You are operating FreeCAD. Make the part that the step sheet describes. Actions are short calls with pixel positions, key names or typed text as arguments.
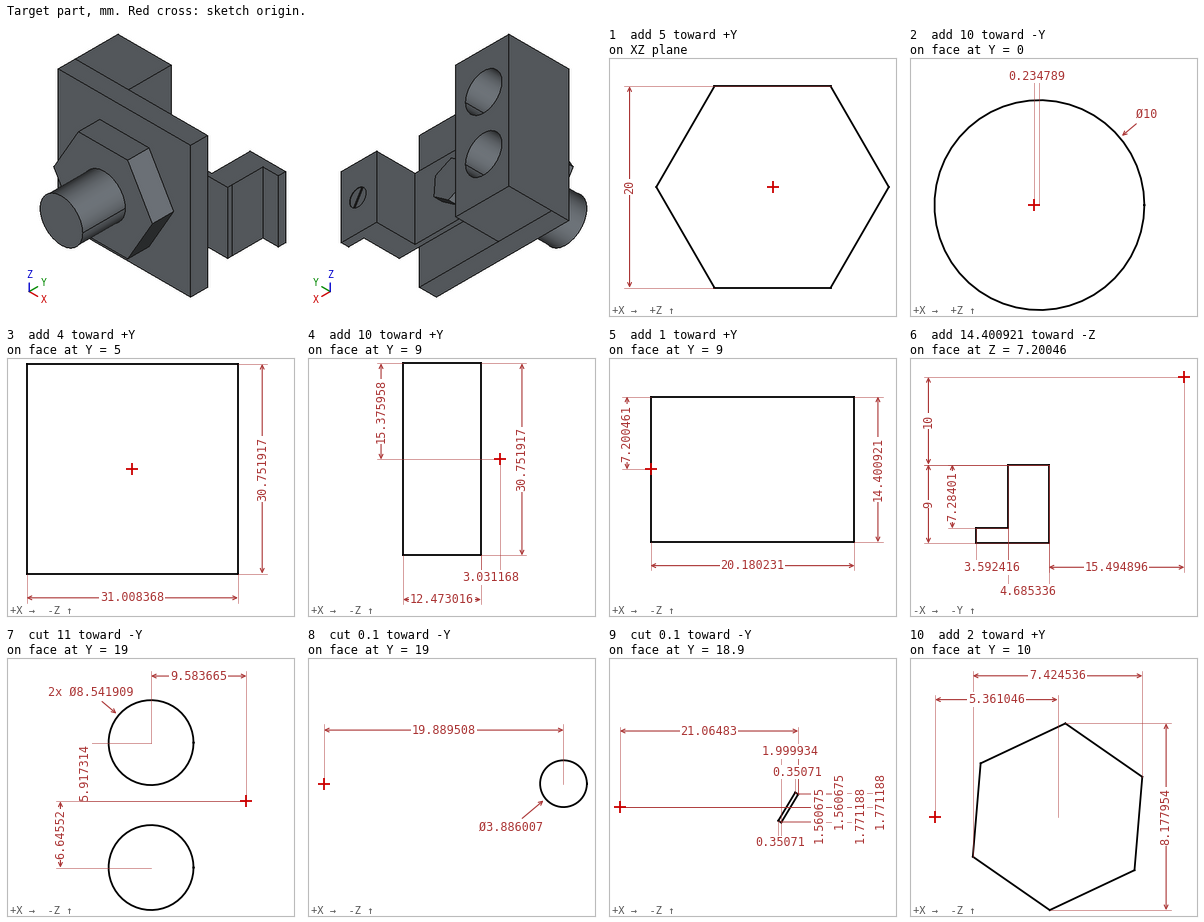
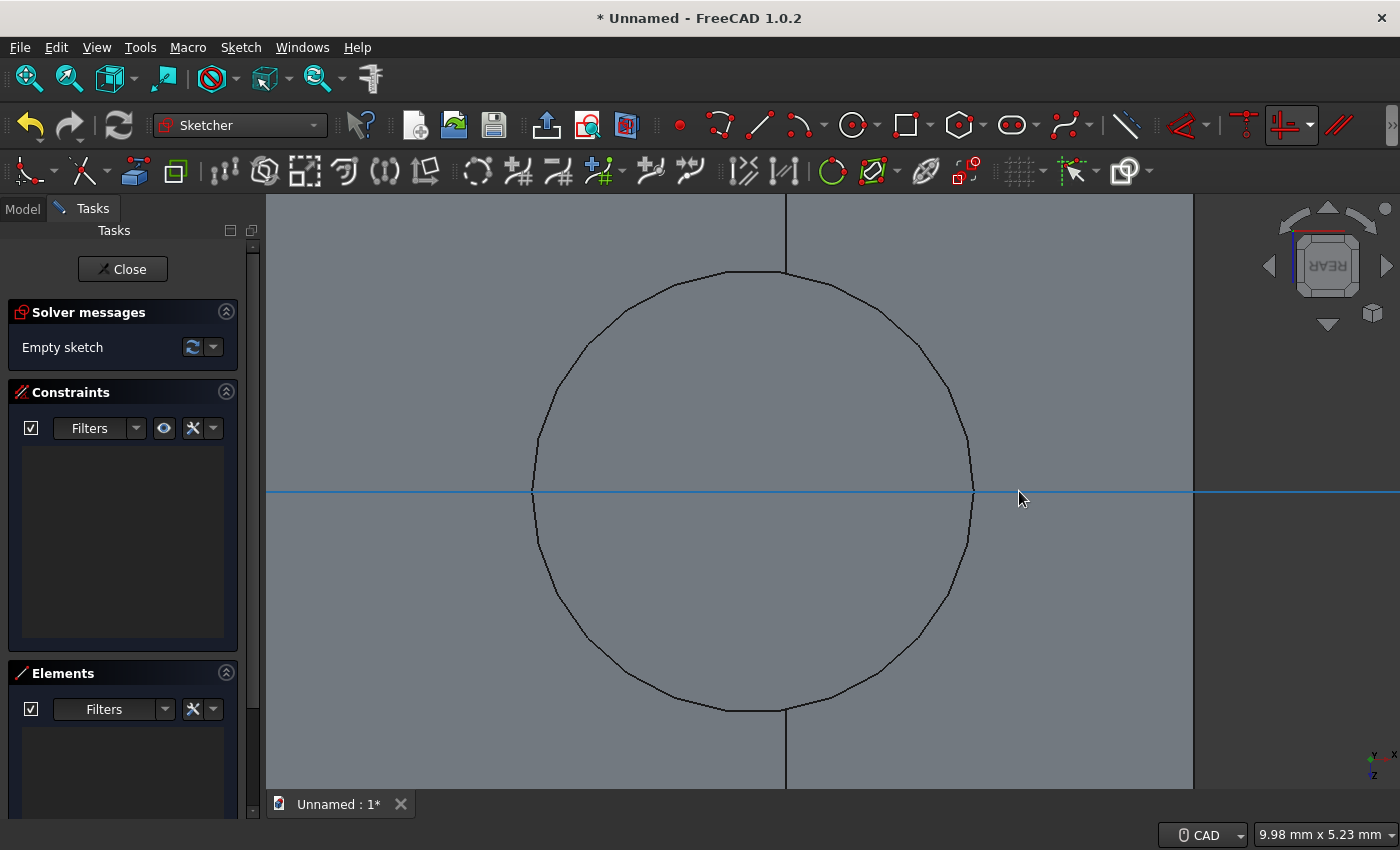
click(720, 126)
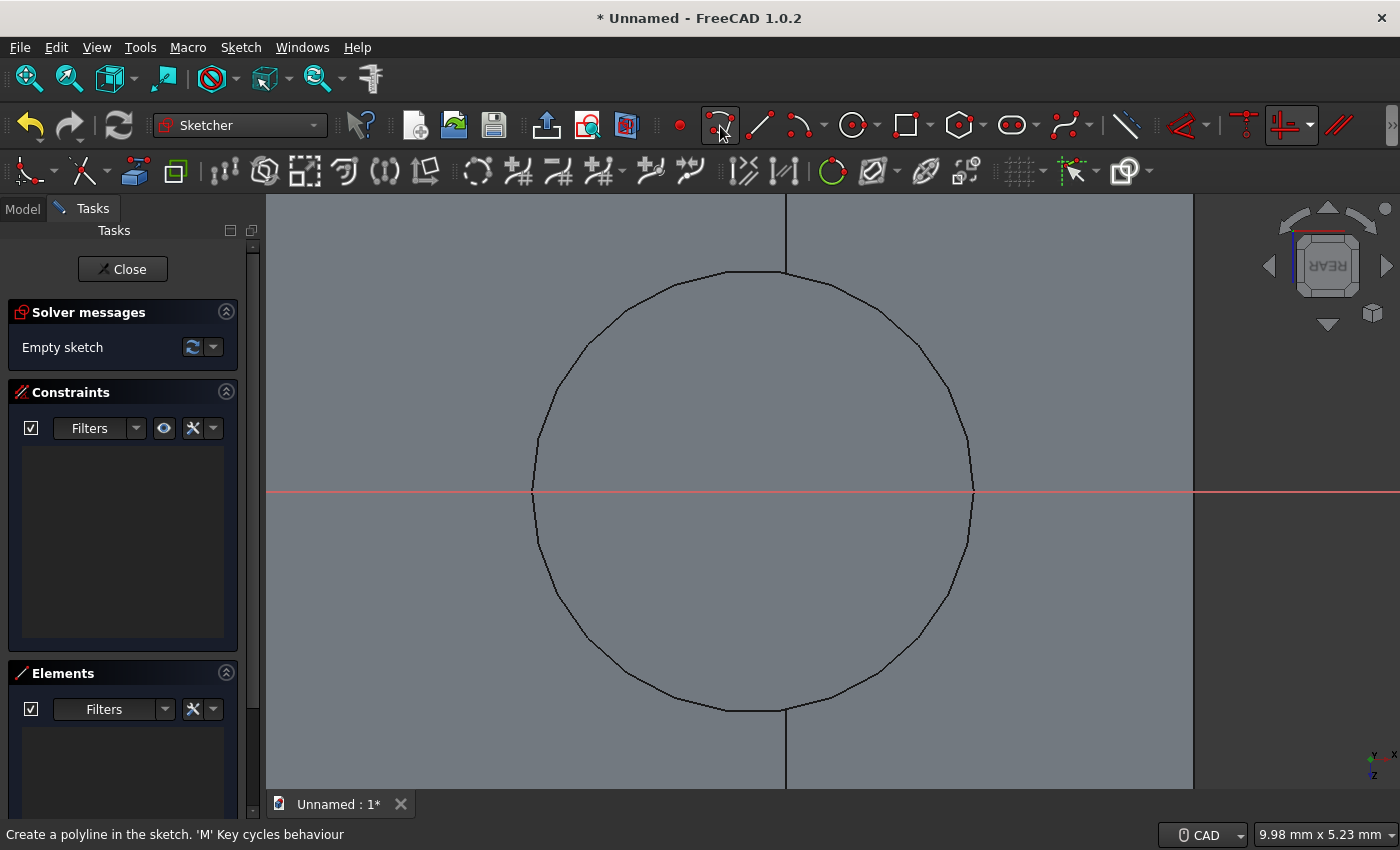
click(619, 669)
click(659, 693)
click(887, 314)
click(847, 290)
click(619, 670)
key(Escape)
key(Escape)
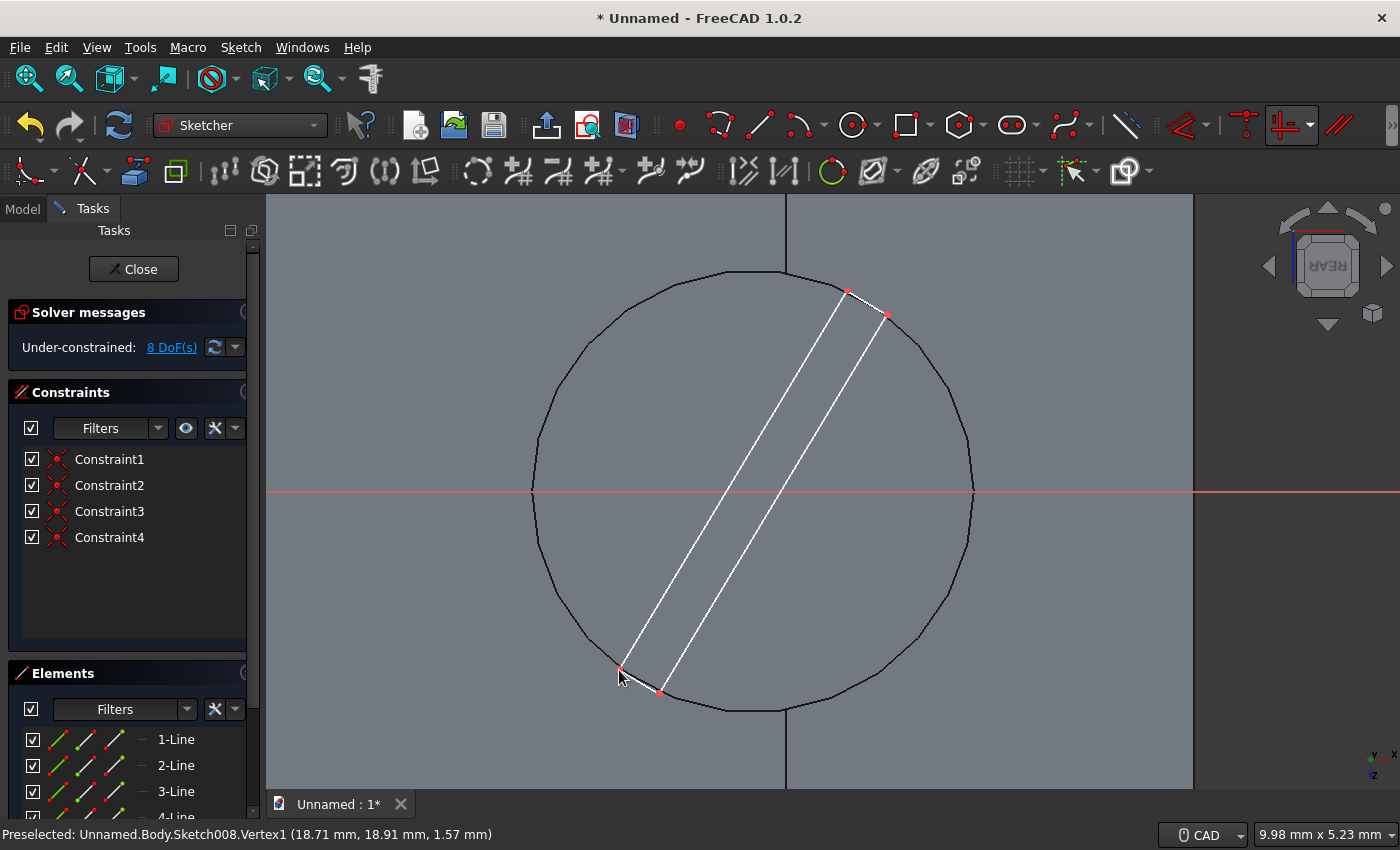
click(1182, 126)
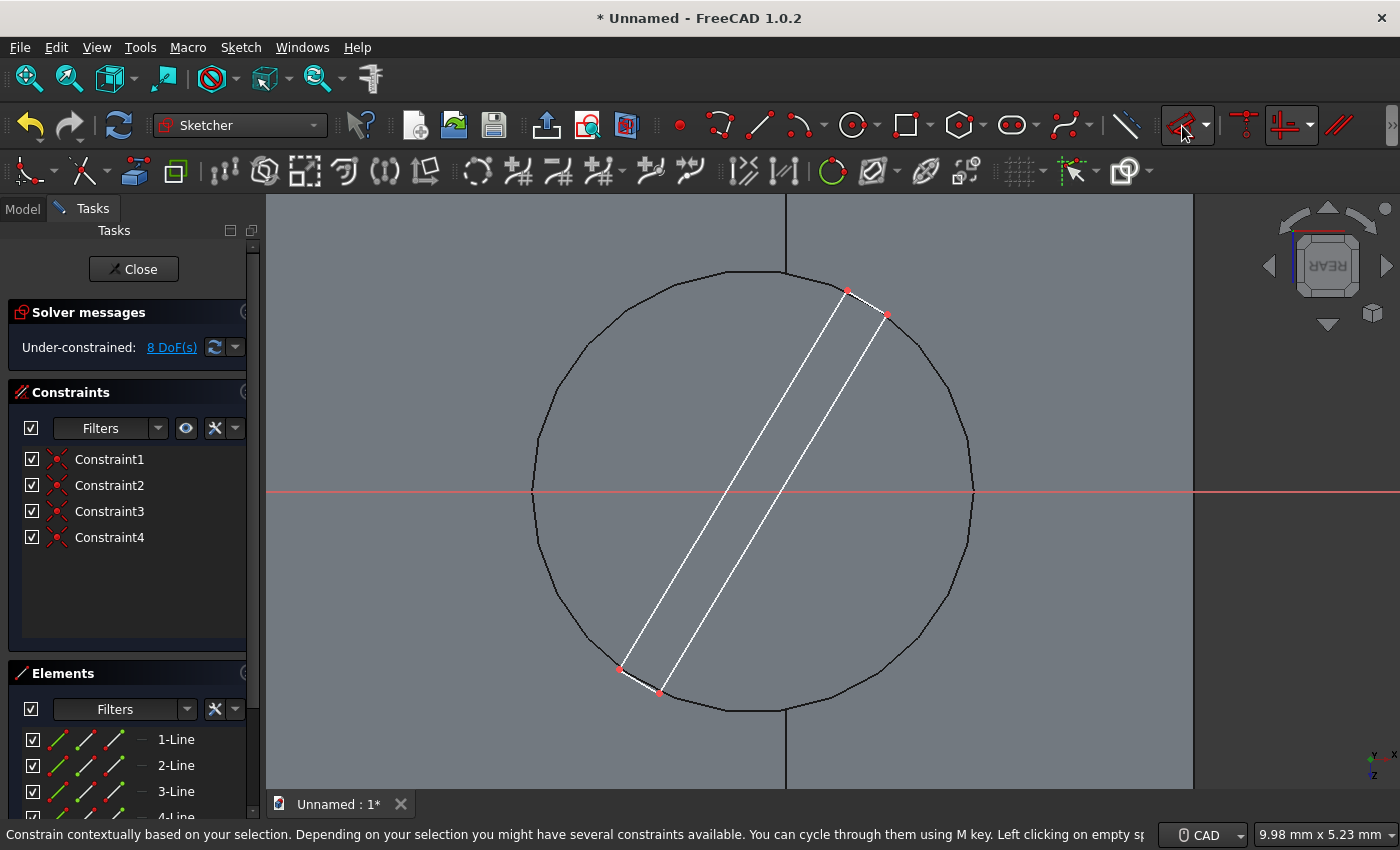
click(631, 677)
click(639, 728)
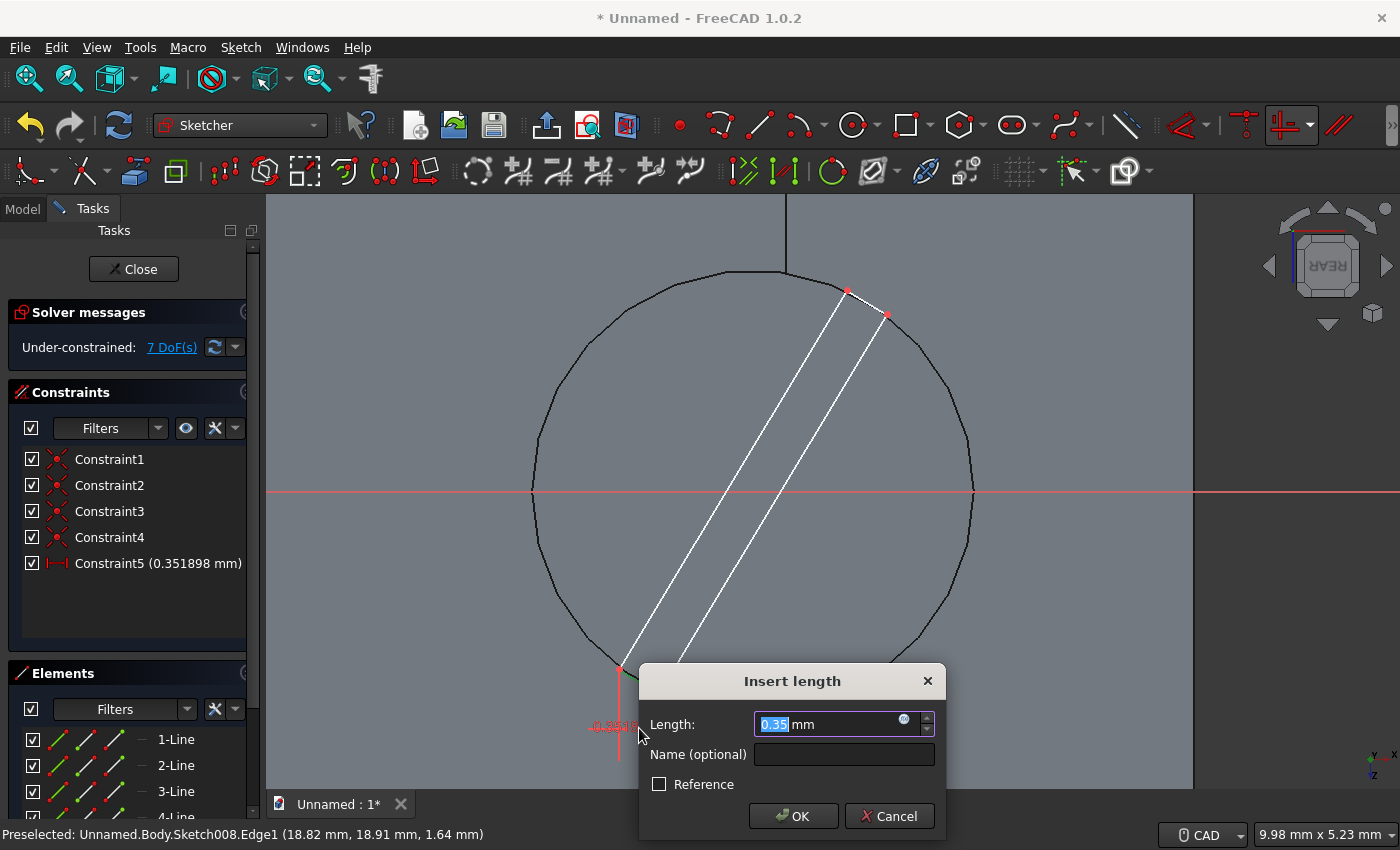
text(0.35071)
key(Return)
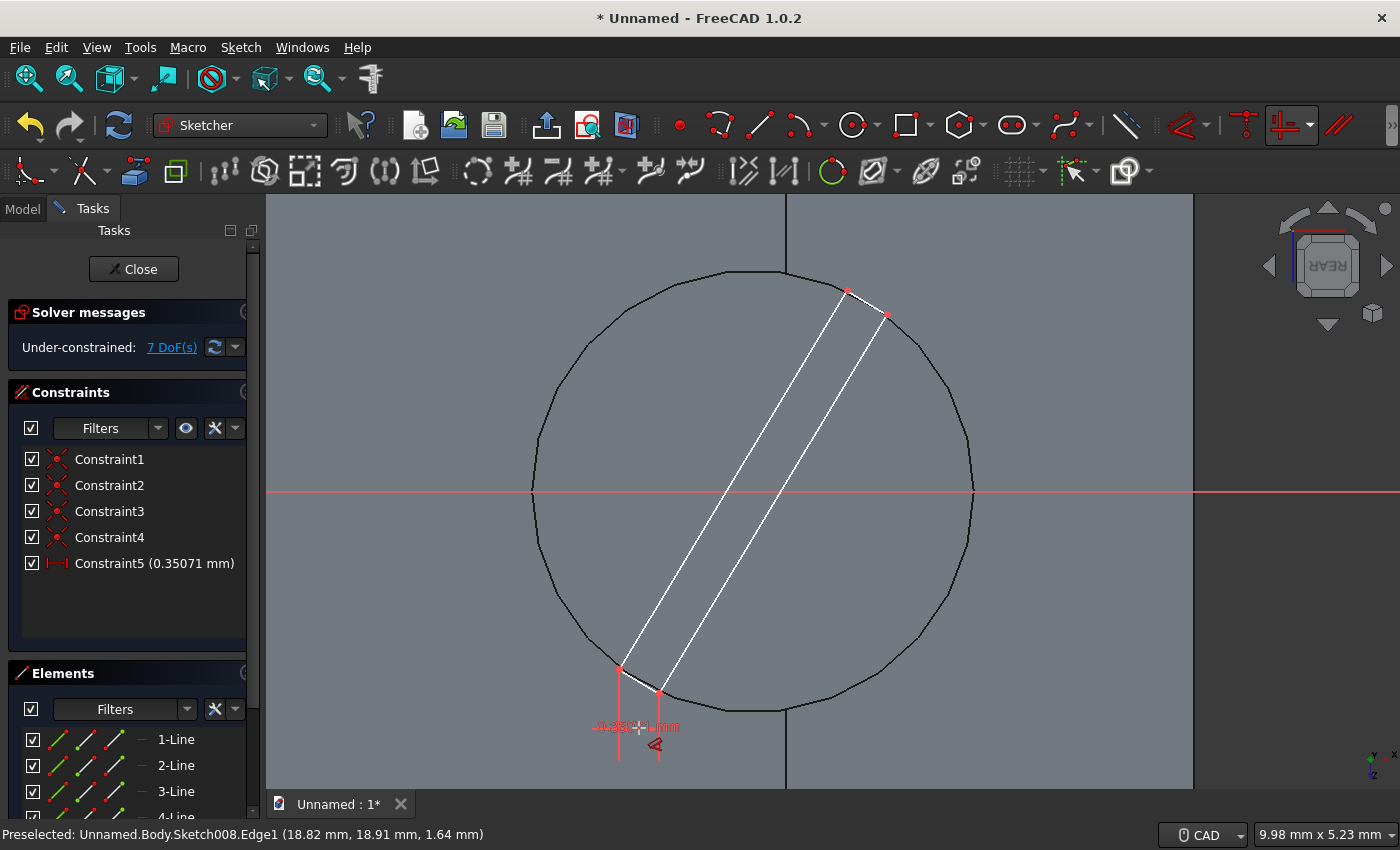
click(875, 308)
click(867, 257)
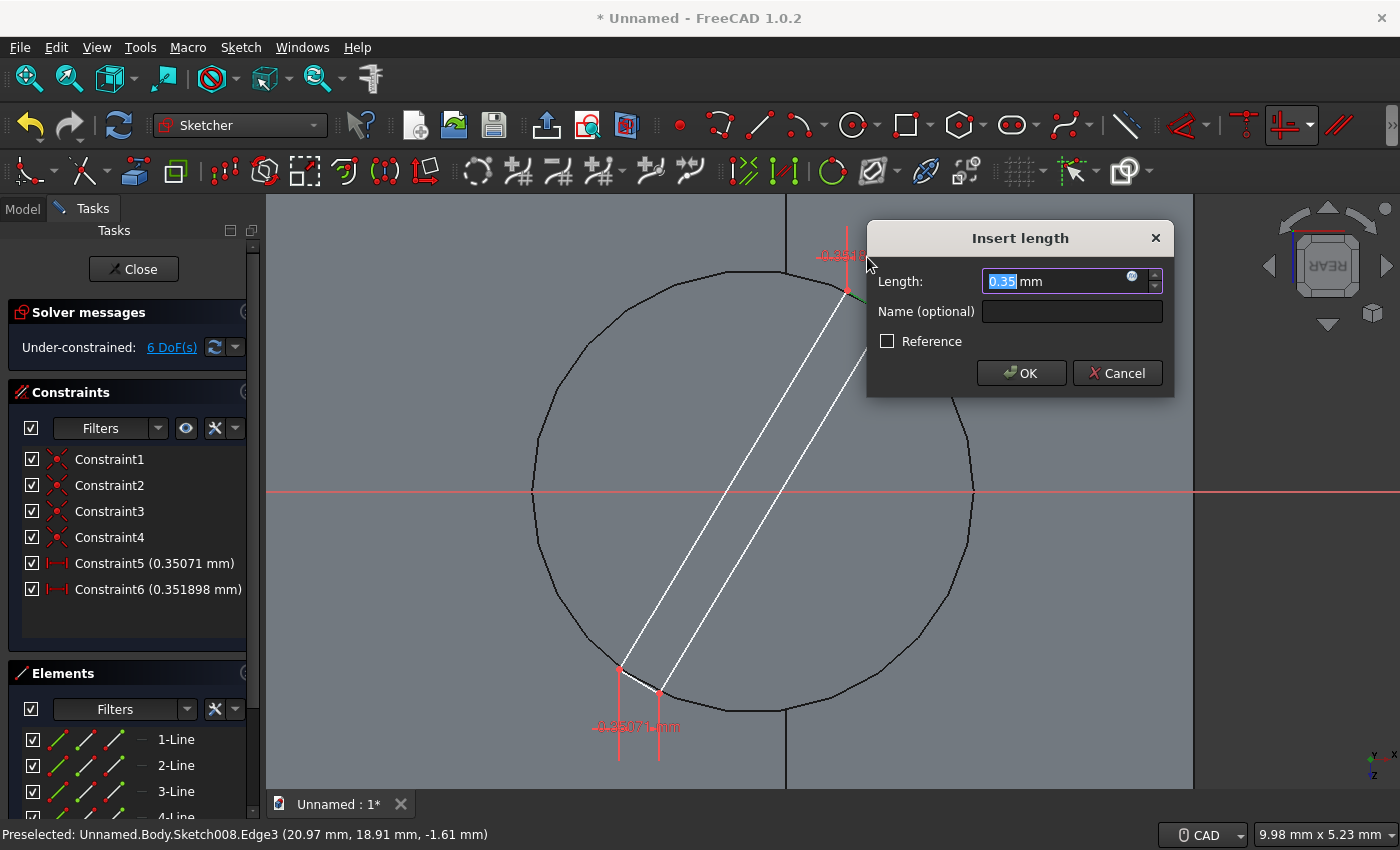
text(0.35071)
key(Return)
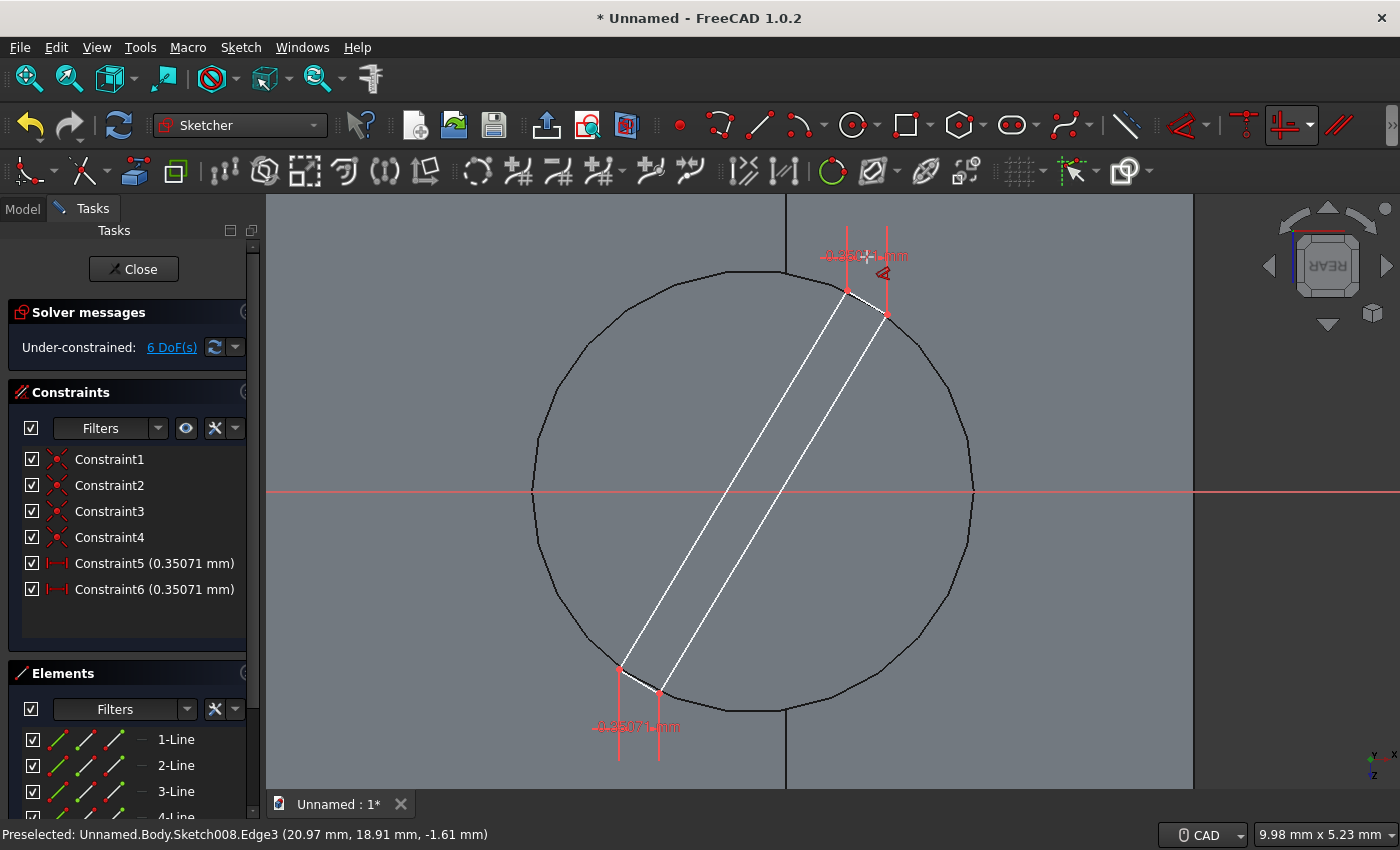
click(619, 670)
click(653, 581)